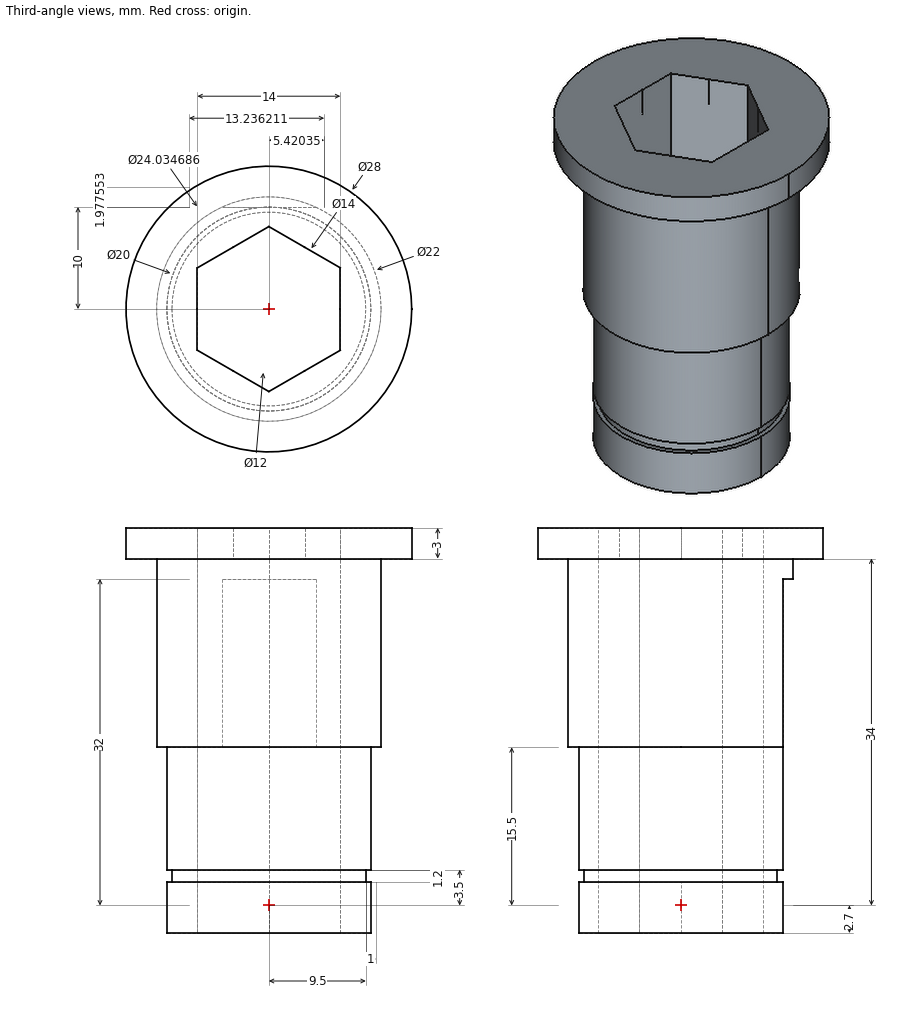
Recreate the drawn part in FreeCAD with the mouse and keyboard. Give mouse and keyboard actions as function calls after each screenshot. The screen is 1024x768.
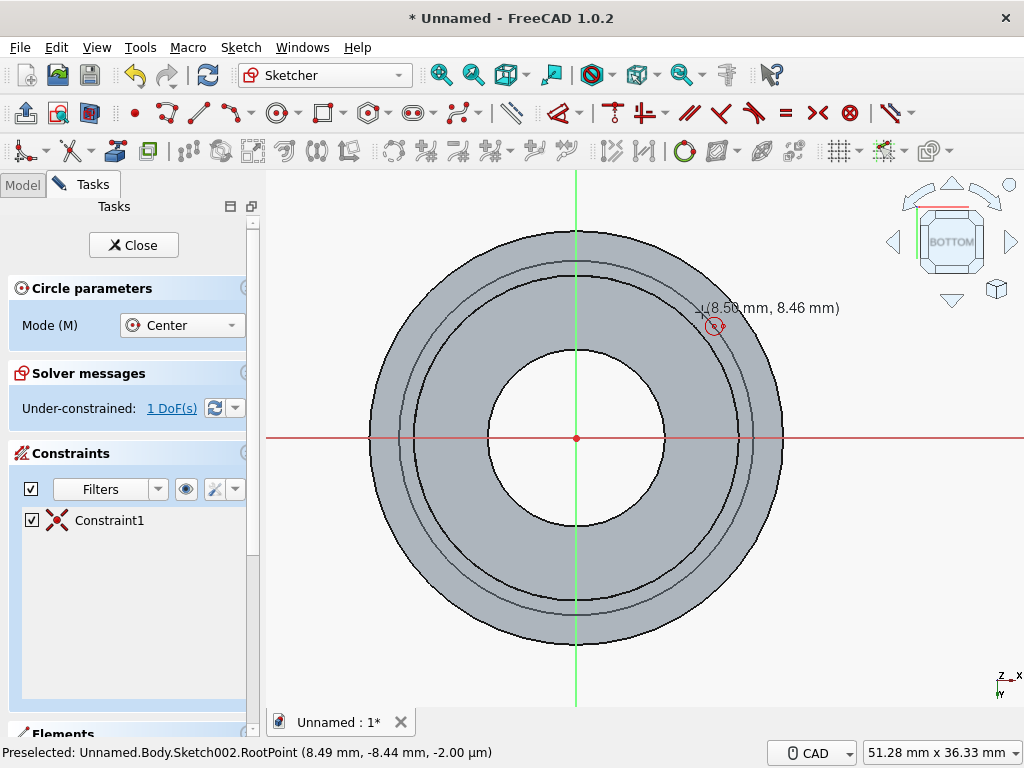
click(576, 438)
click(681, 333)
key(Escape)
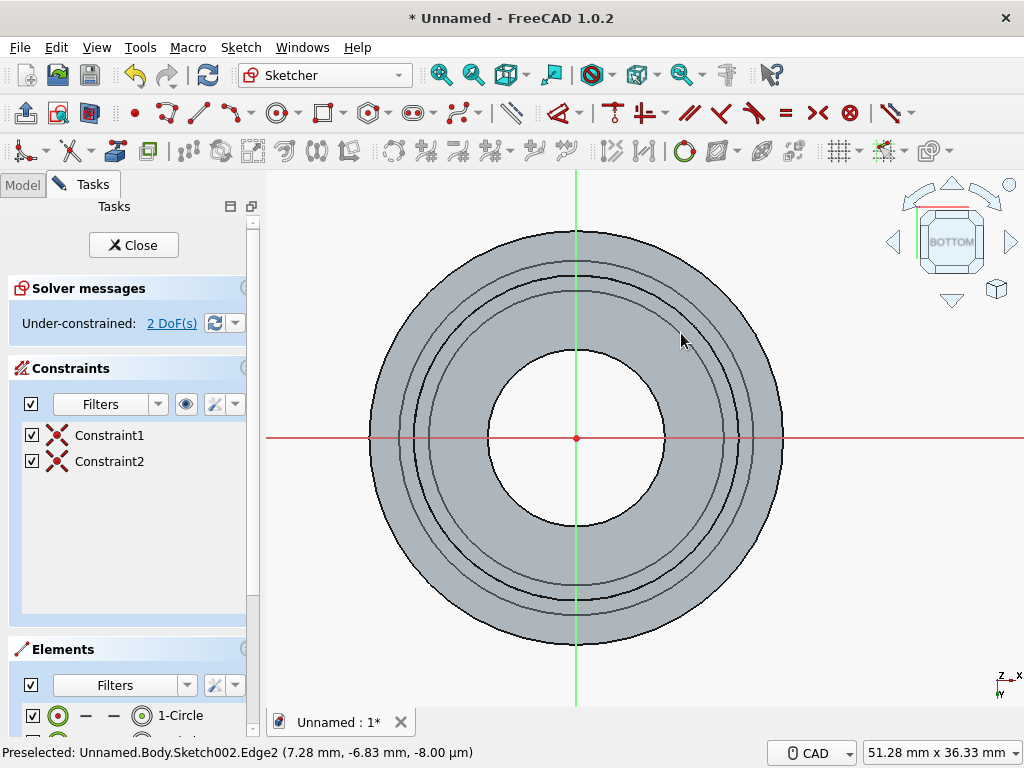
click(558, 114)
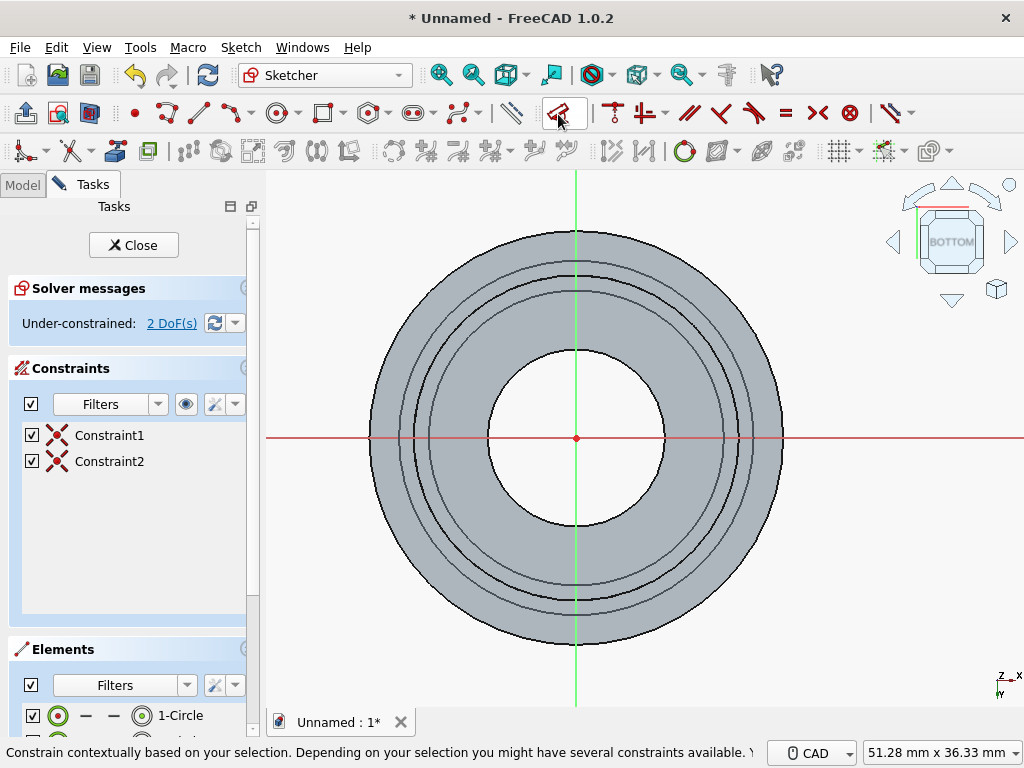
click(701, 312)
click(724, 289)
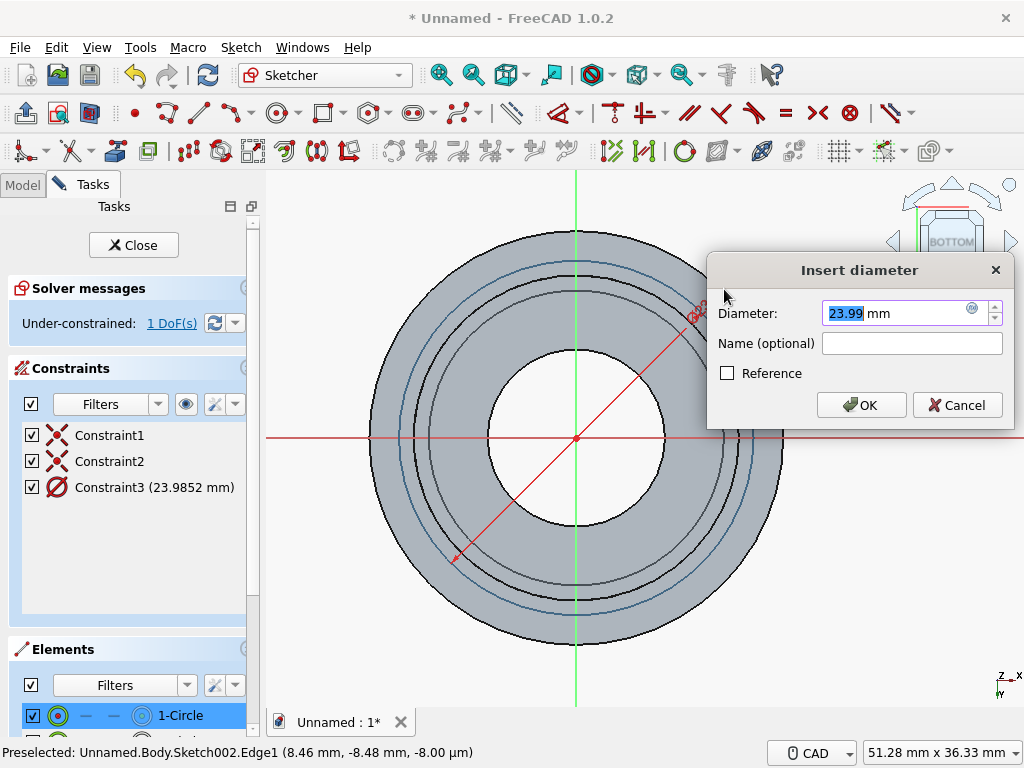
text(24.034686)
key(Return)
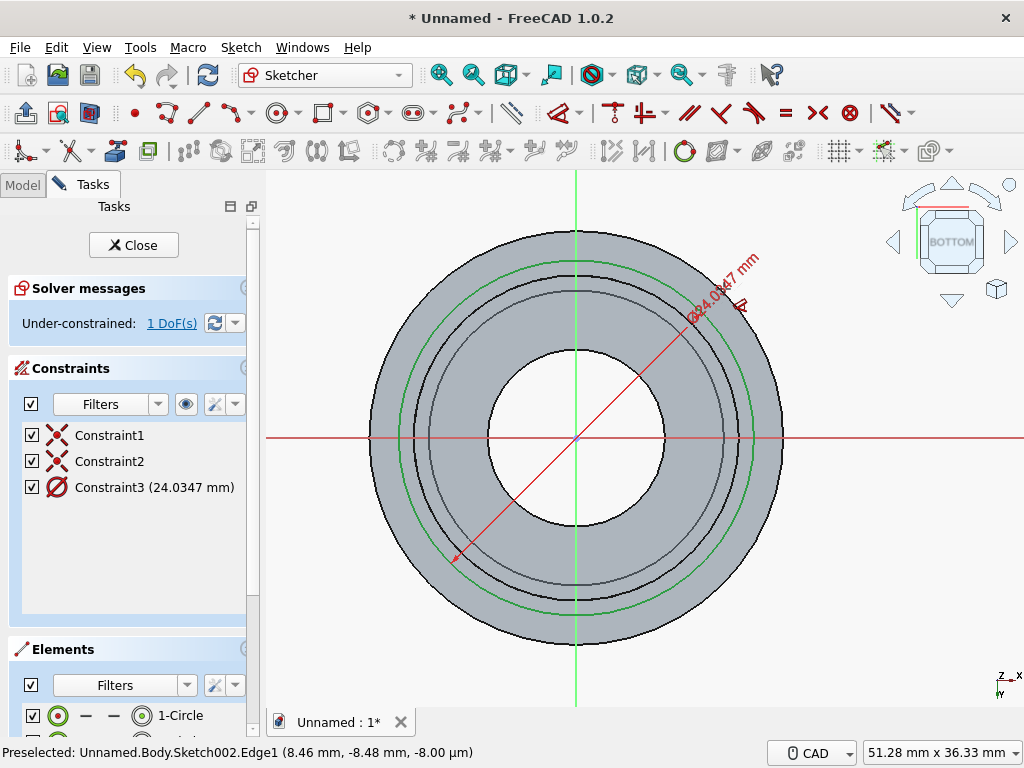
click(680, 333)
click(770, 380)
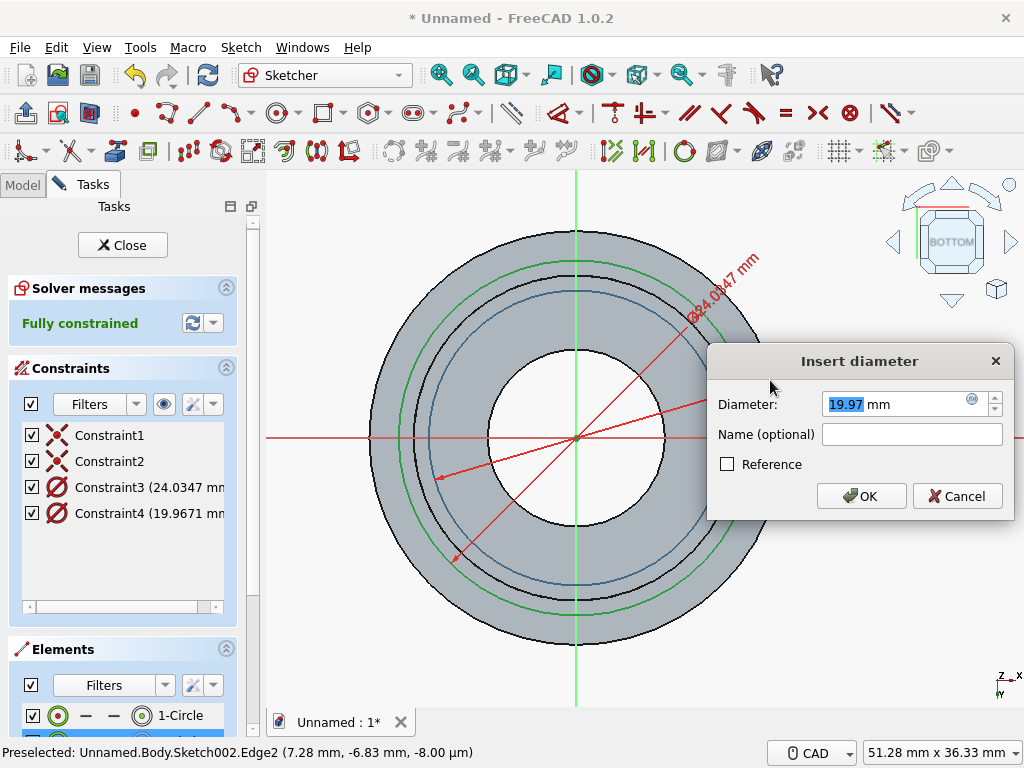
text(20)
key(Return)
key(Escape)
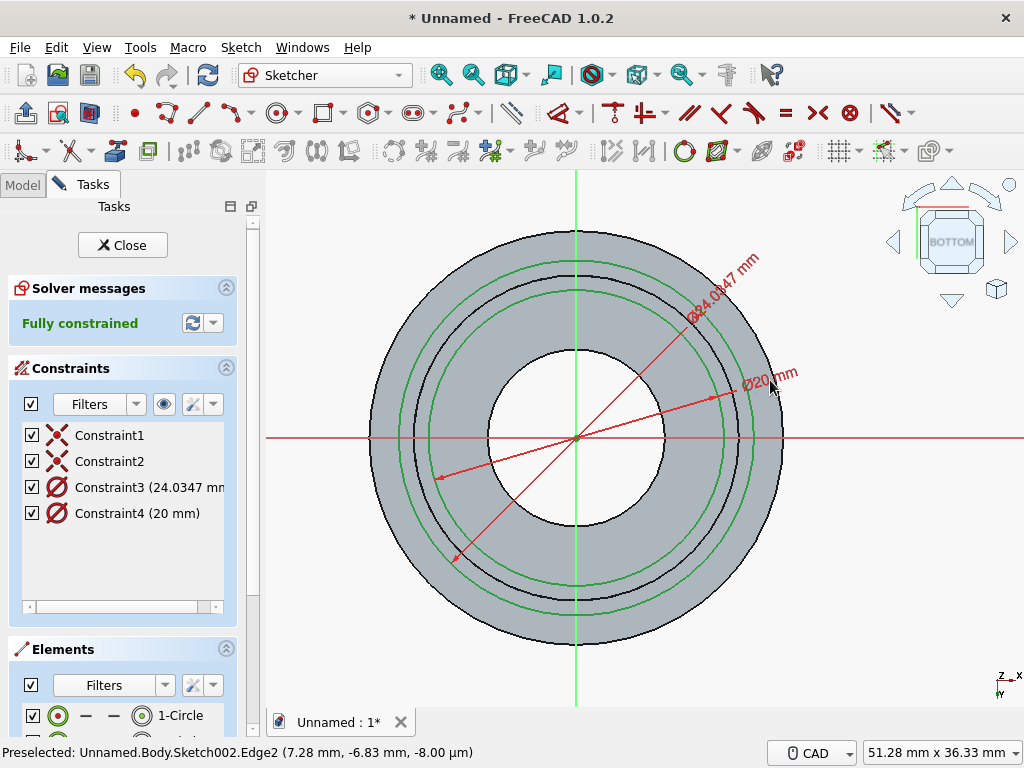
click(123, 245)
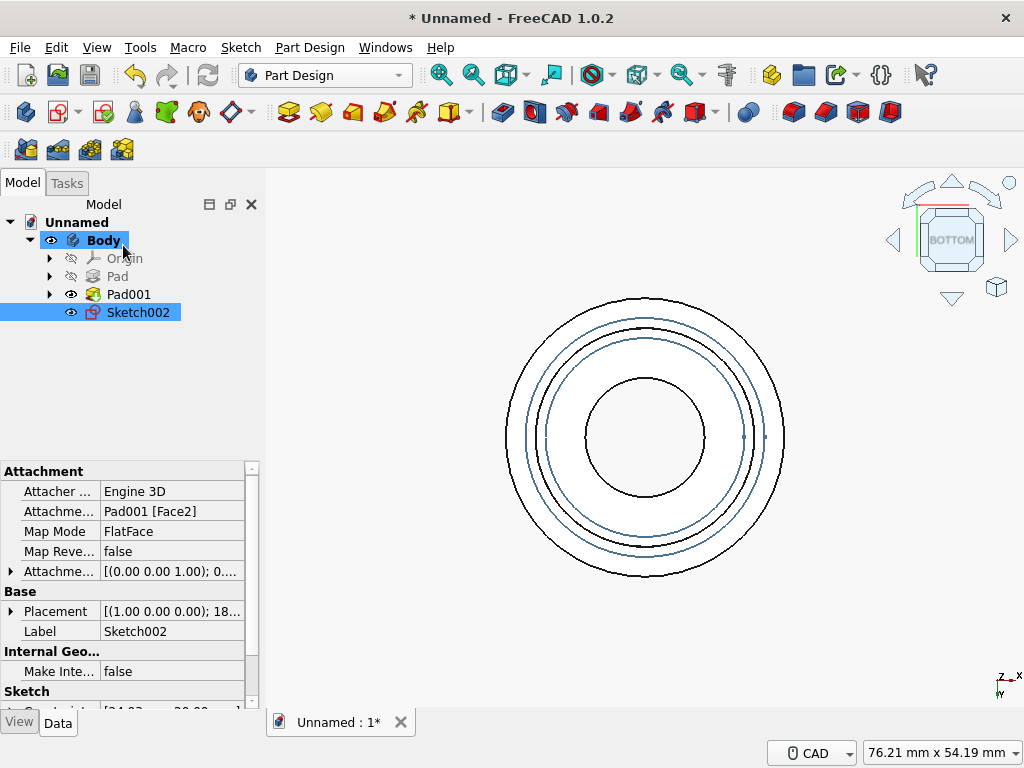
click(504, 112)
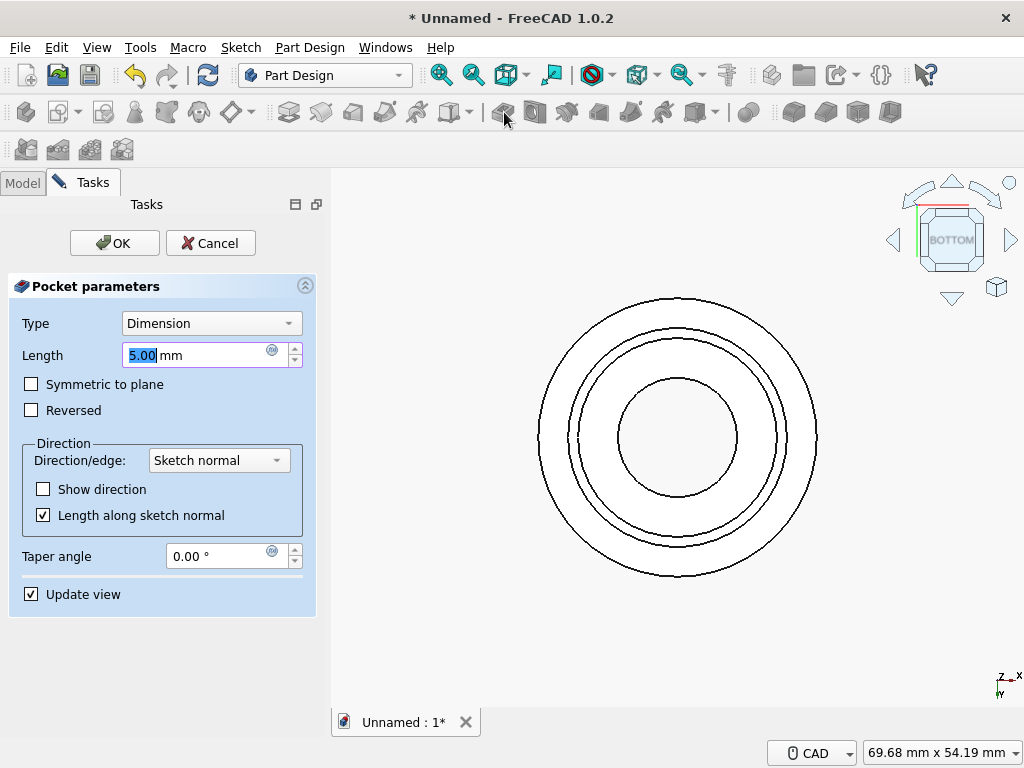
text(15.5)
key(Tab)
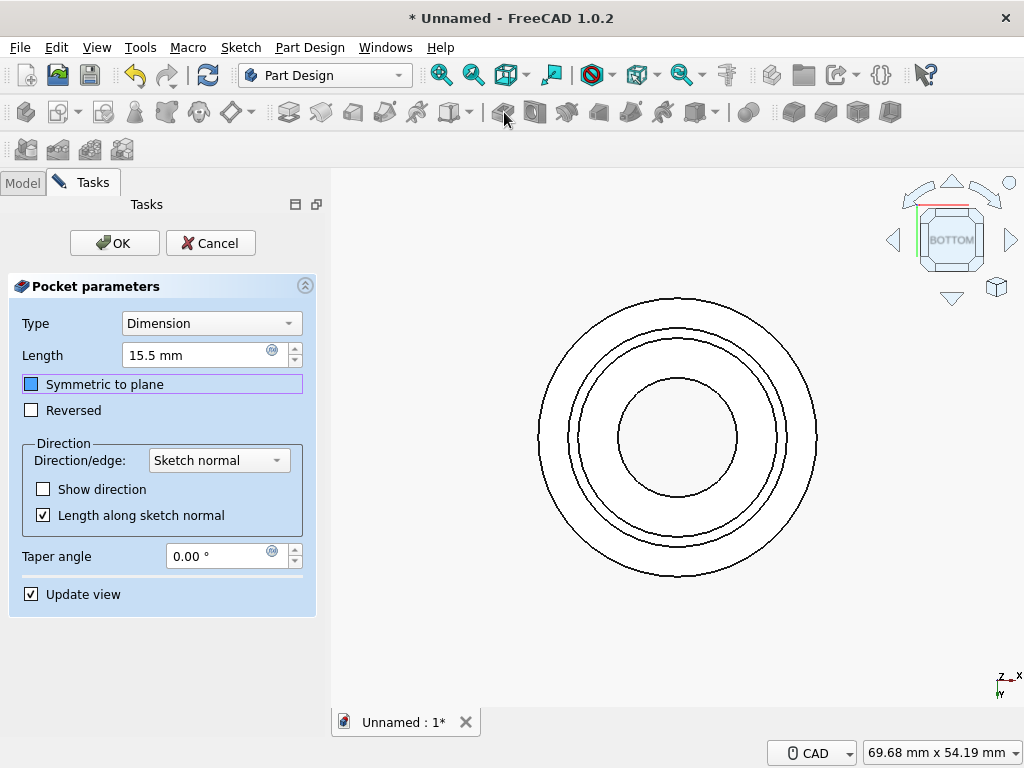
click(115, 243)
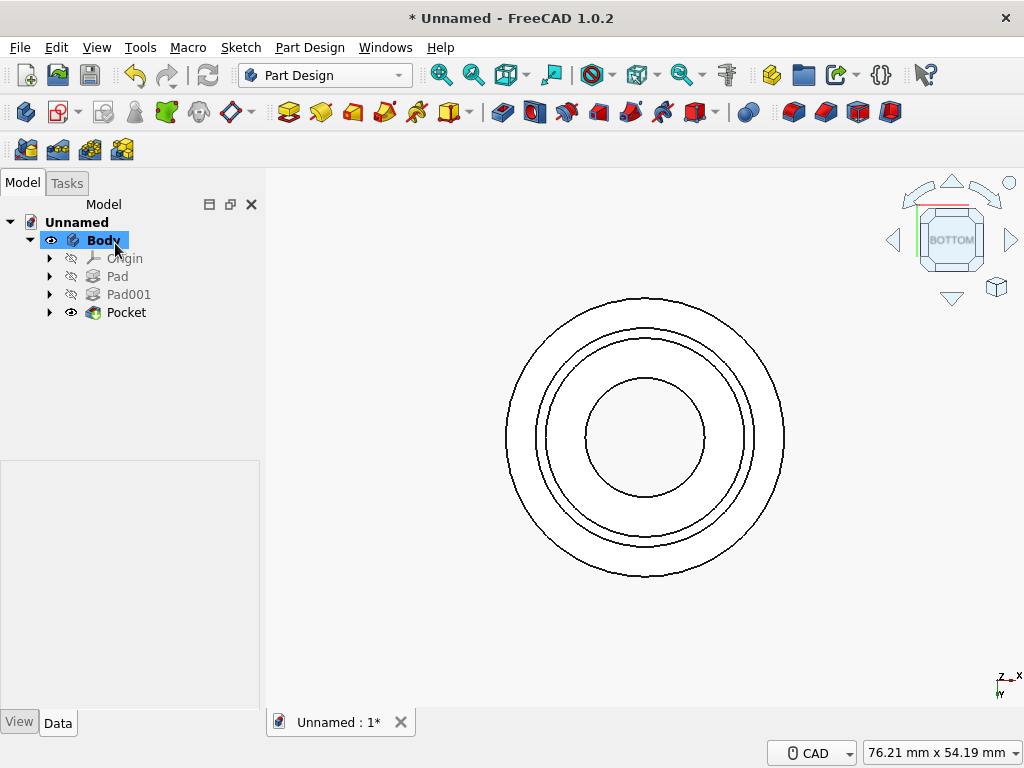
click(58, 112)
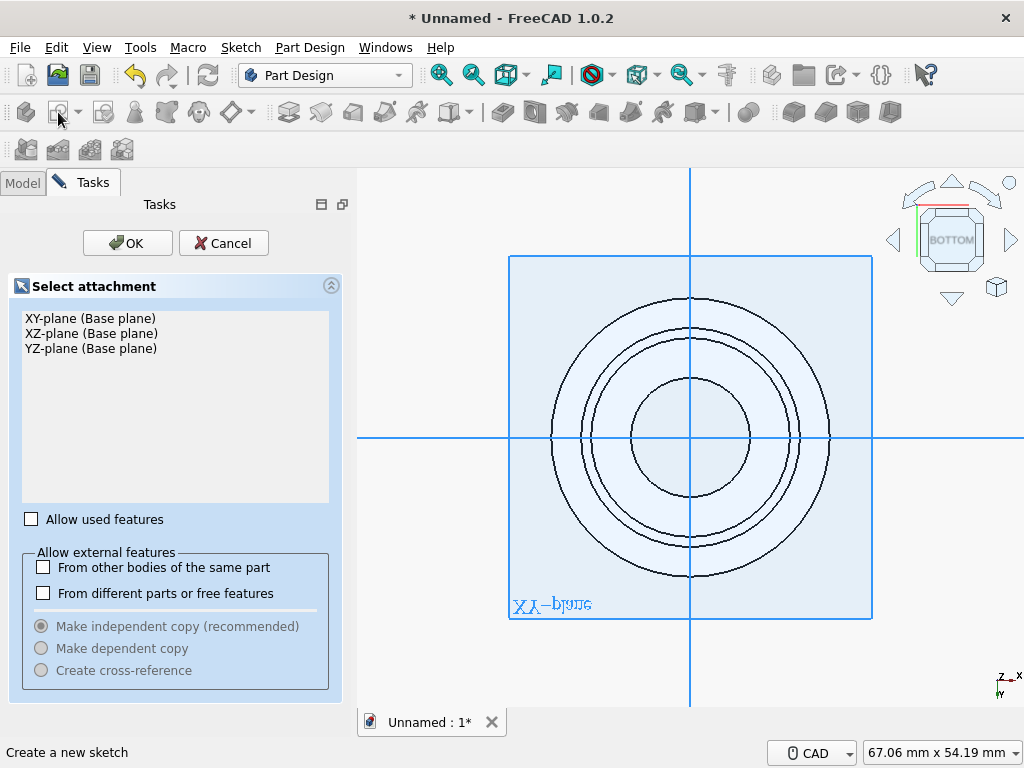
click(82, 318)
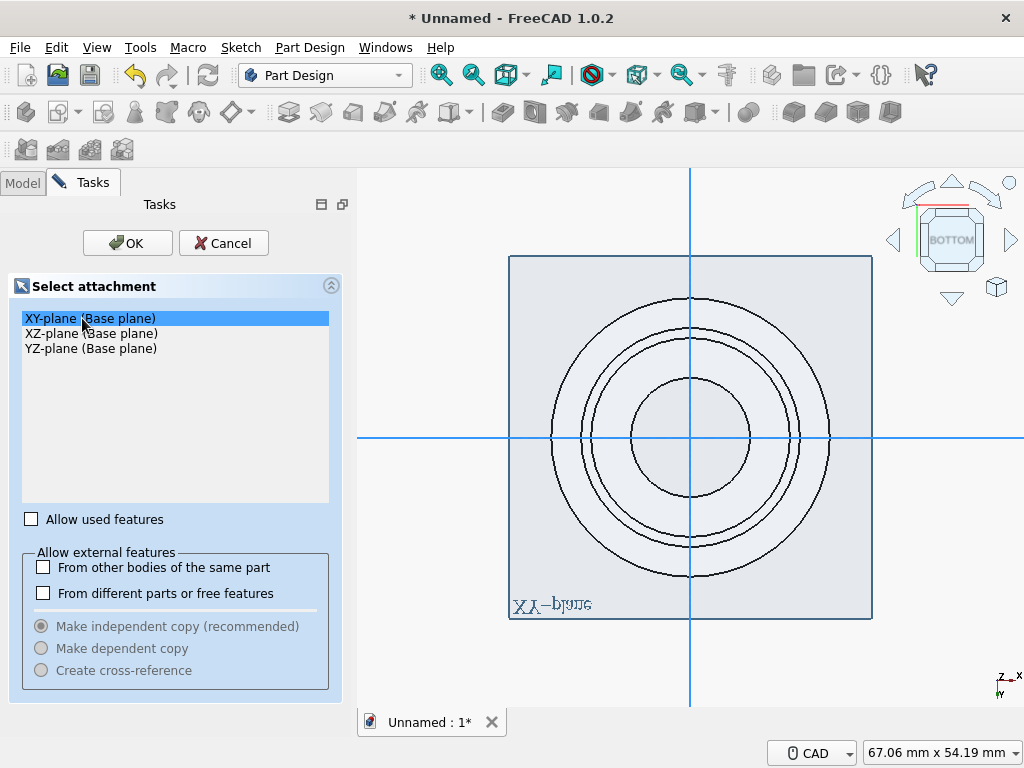
click(128, 243)